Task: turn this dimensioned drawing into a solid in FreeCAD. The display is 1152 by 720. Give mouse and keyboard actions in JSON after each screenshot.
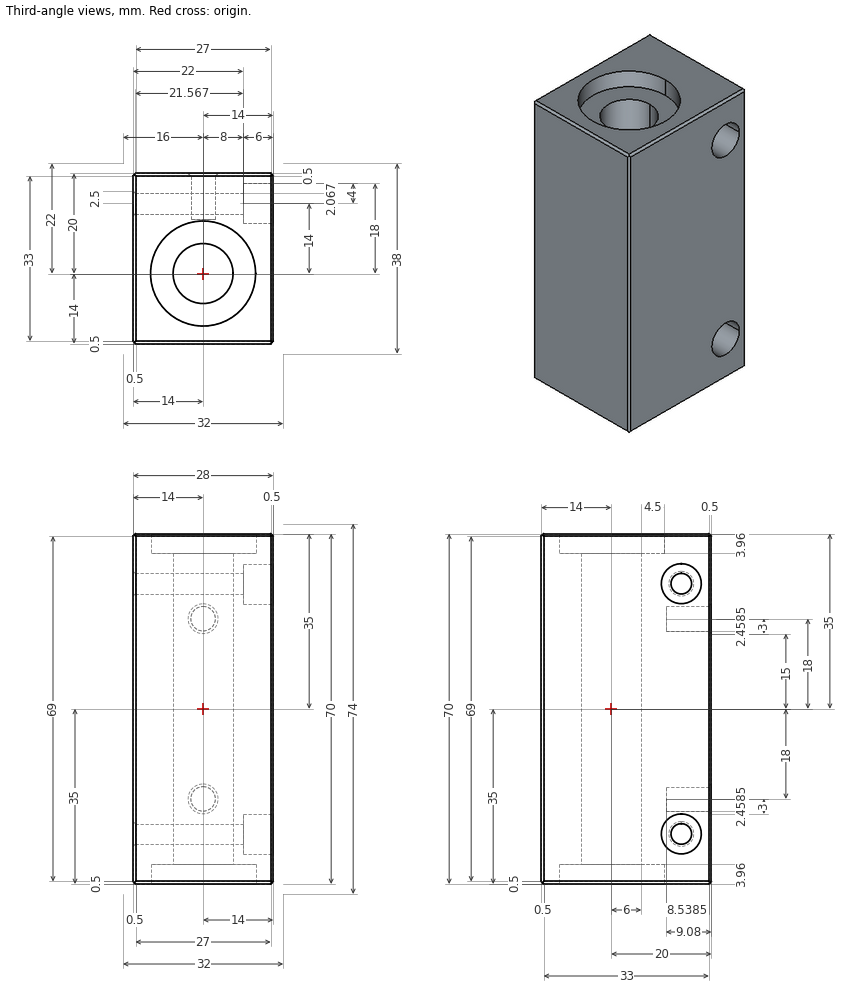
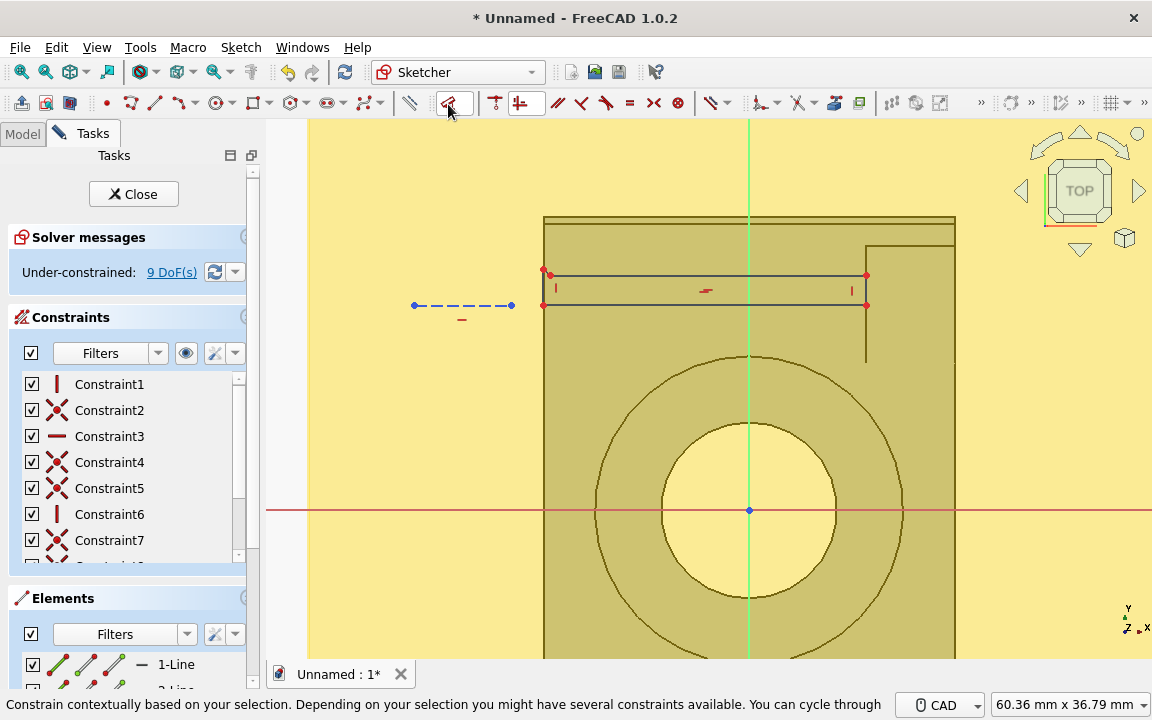
{"action": "left_click", "coordinate": [640, 305]}
{"action": "left_click", "coordinate": [705, 339]}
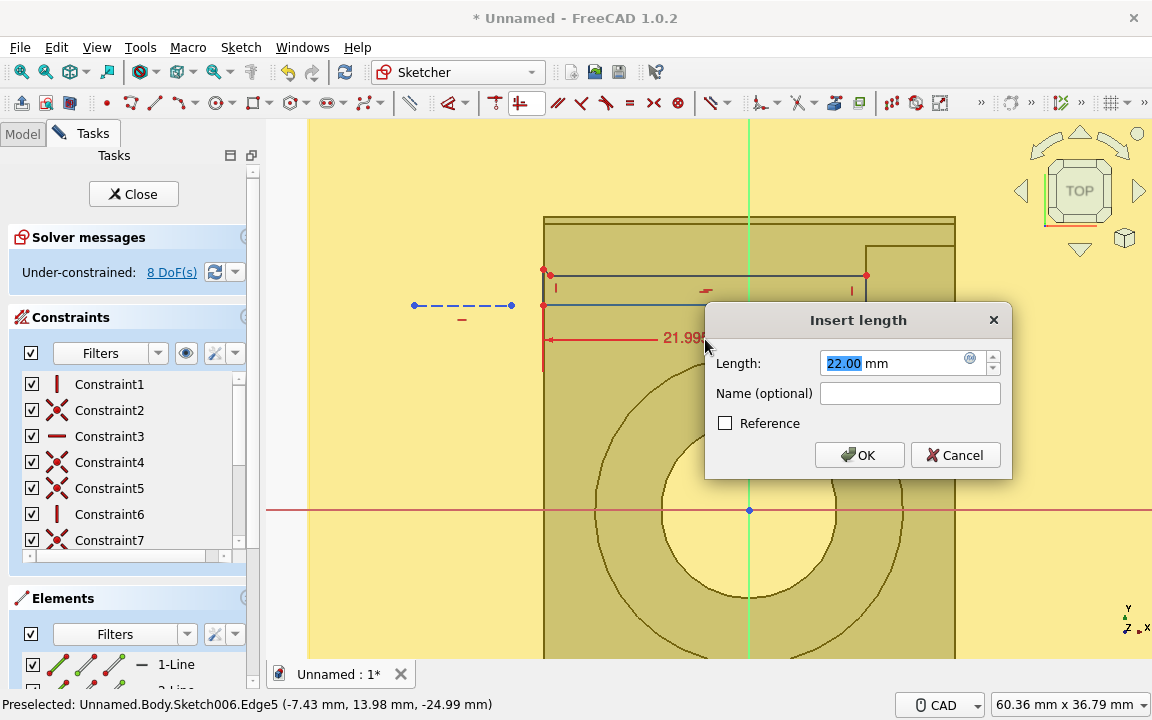
{"action": "type", "text": "22"}
{"action": "key", "text": "Return"}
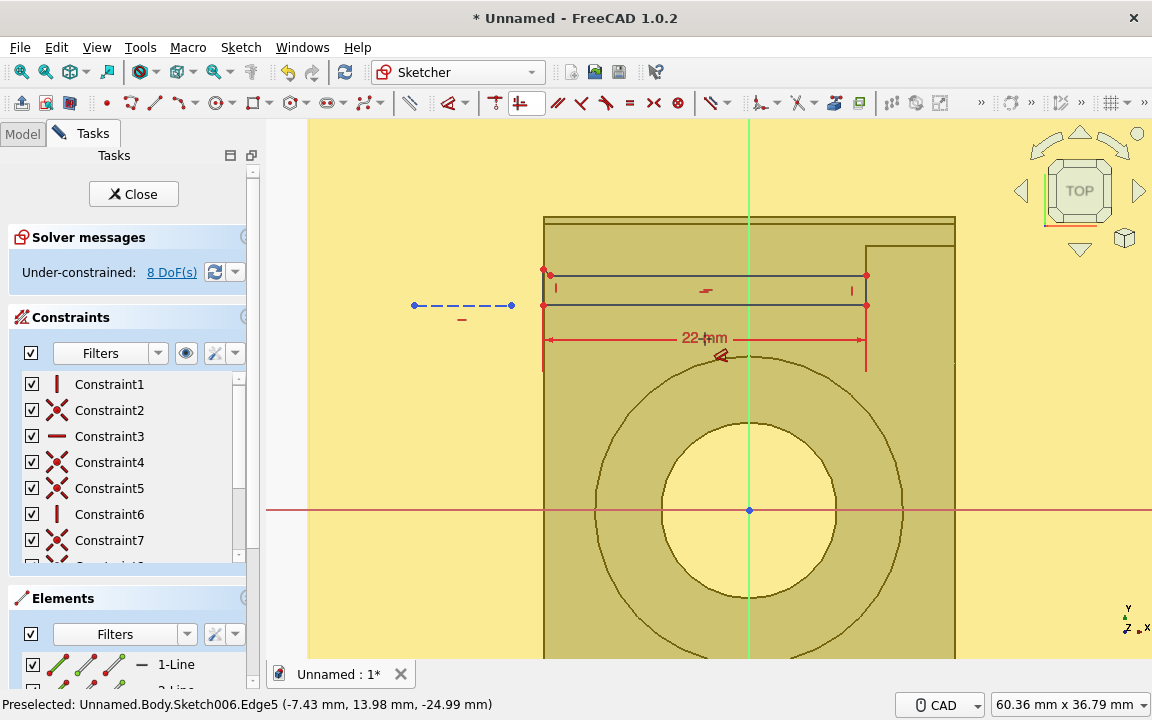
{"action": "left_click", "coordinate": [866, 305]}
{"action": "left_click", "coordinate": [808, 544]}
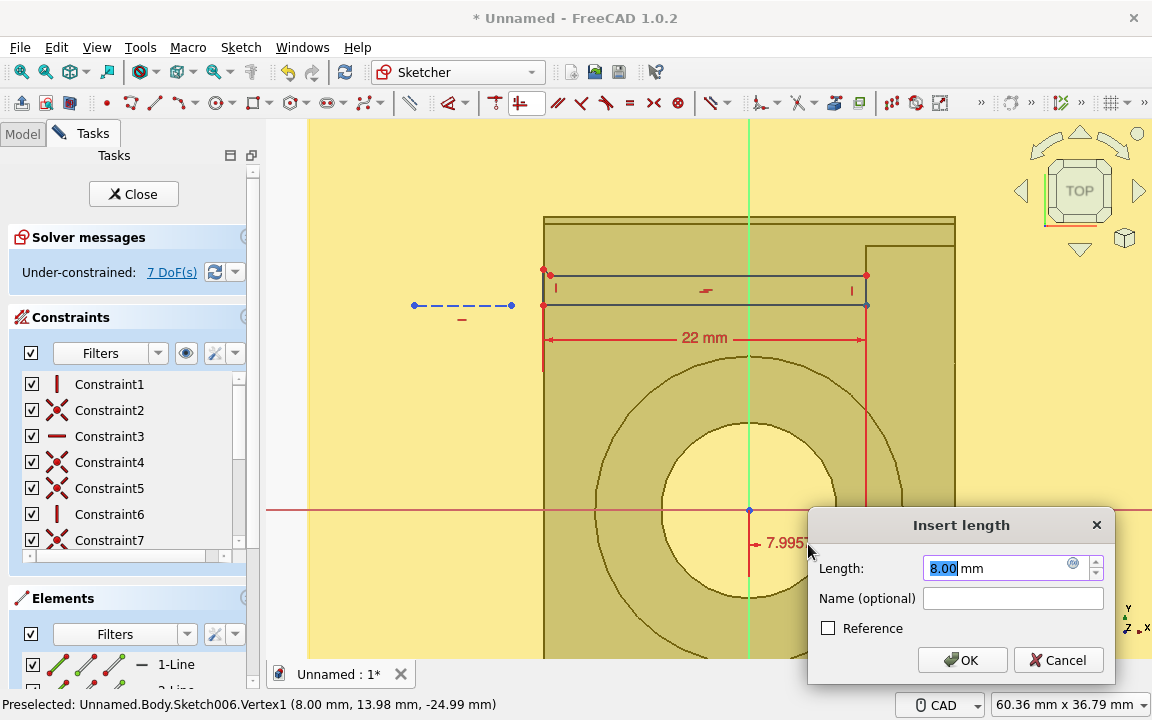
{"action": "type", "text": "8"}
{"action": "key", "text": "Return"}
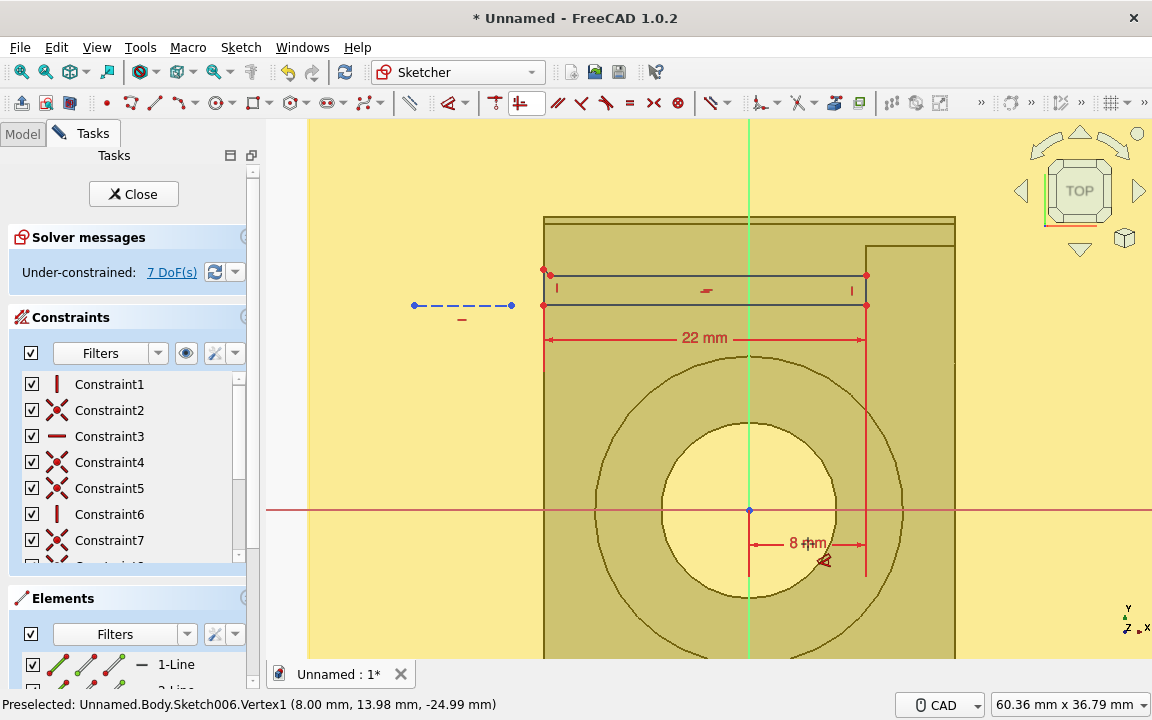
{"action": "scroll", "coordinate": [544, 294], "scroll_direction": "up", "scroll_amount": 2}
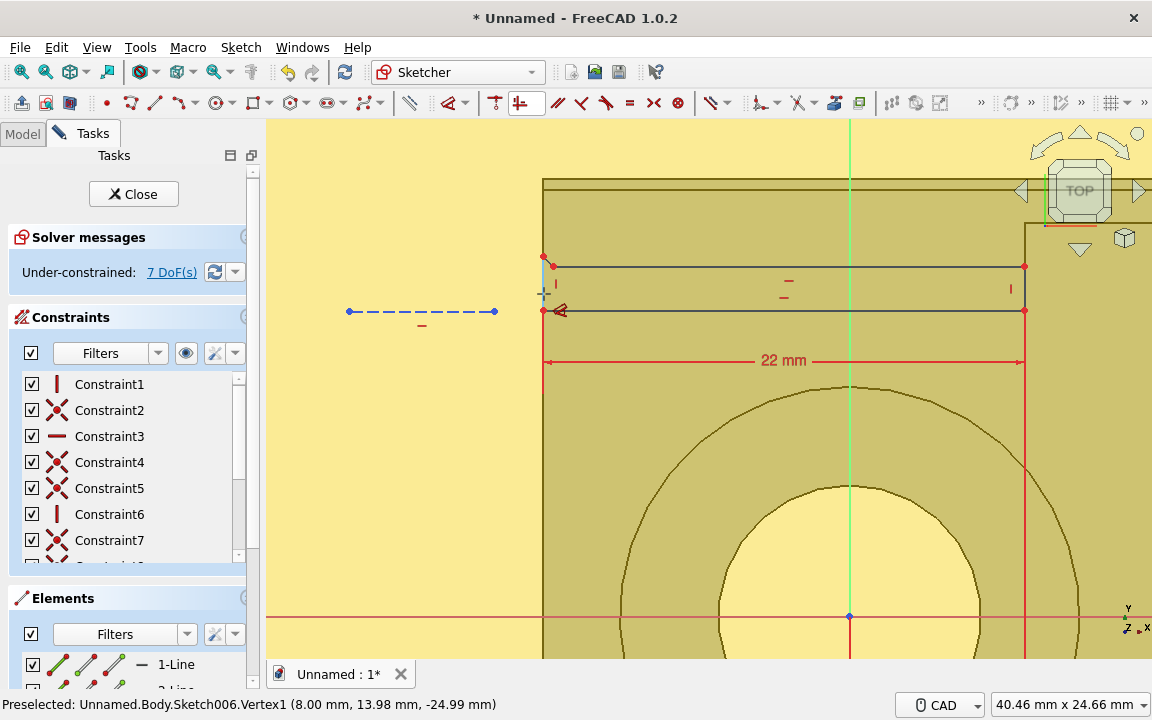
{"action": "left_click", "coordinate": [543, 294]}
{"action": "left_click", "coordinate": [509, 284]}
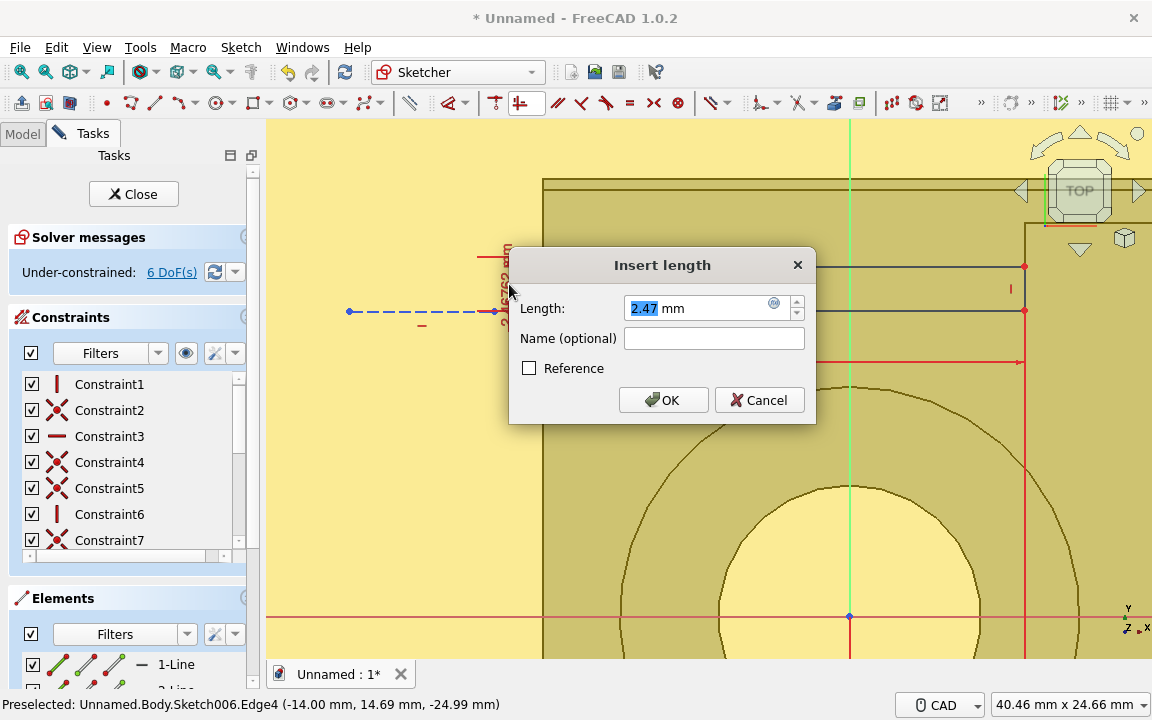
{"action": "type", "text": "2.5"}
{"action": "key", "text": "Return"}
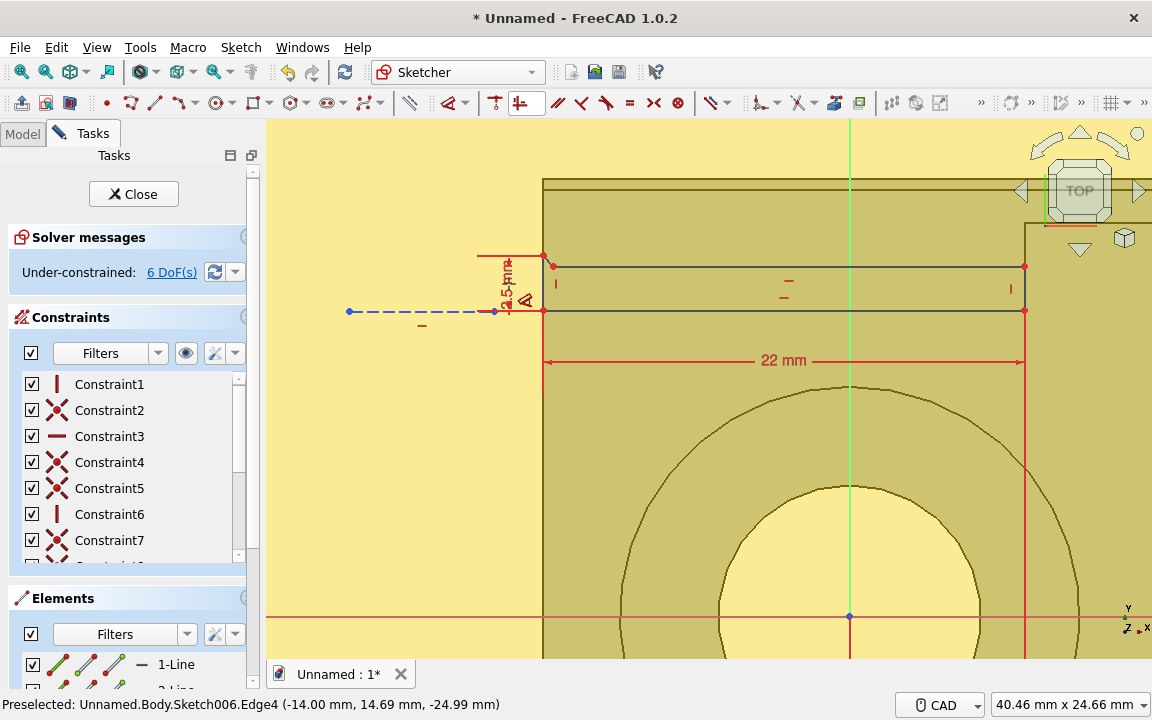
{"action": "scroll", "coordinate": [545, 293], "scroll_direction": "down", "scroll_amount": 2}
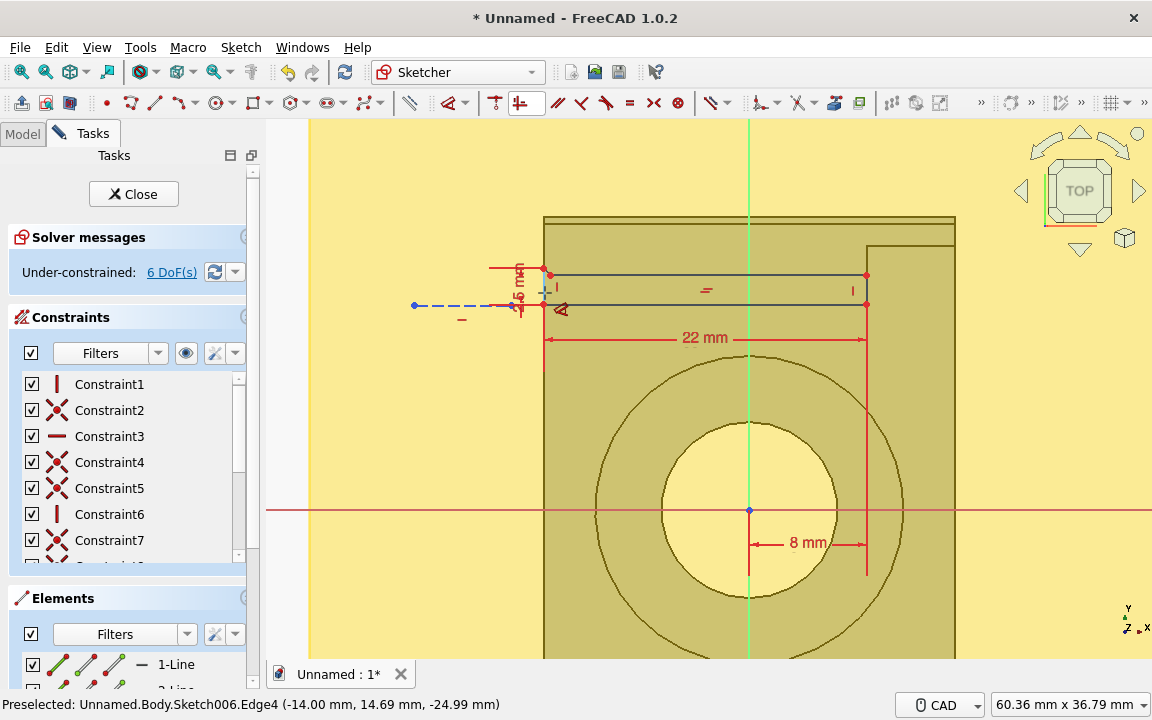
{"action": "left_click", "coordinate": [867, 305]}
{"action": "left_click", "coordinate": [901, 408]}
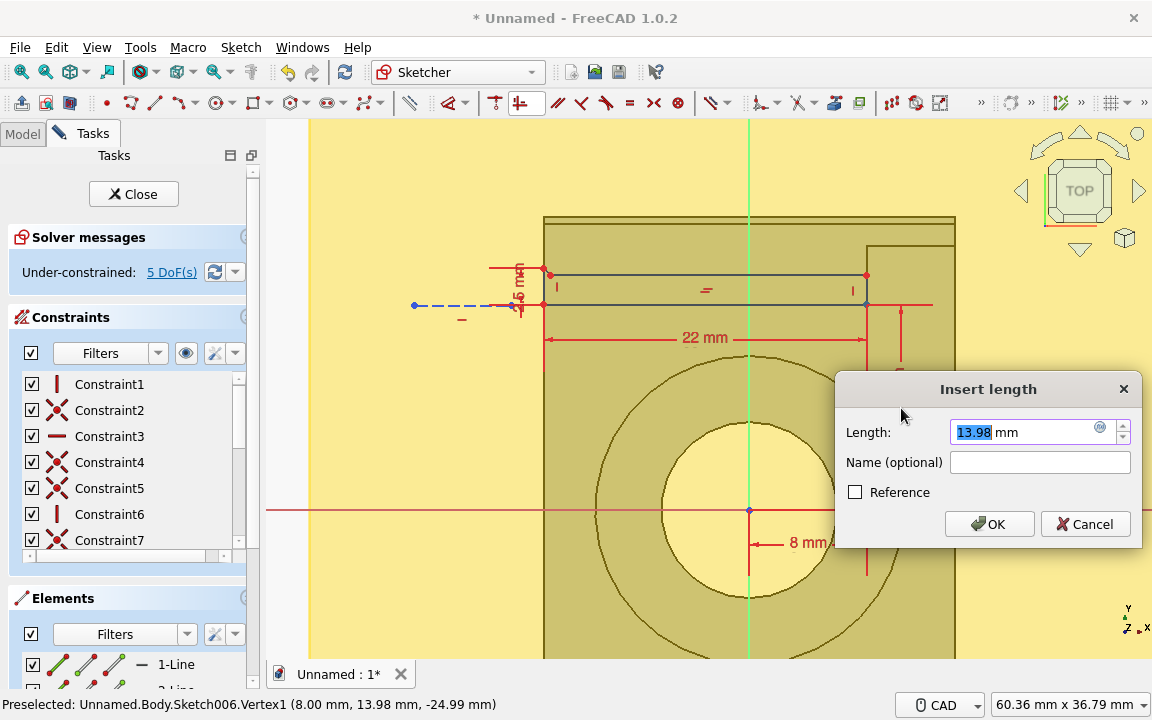
{"action": "type", "text": "14"}
{"action": "key", "text": "Return"}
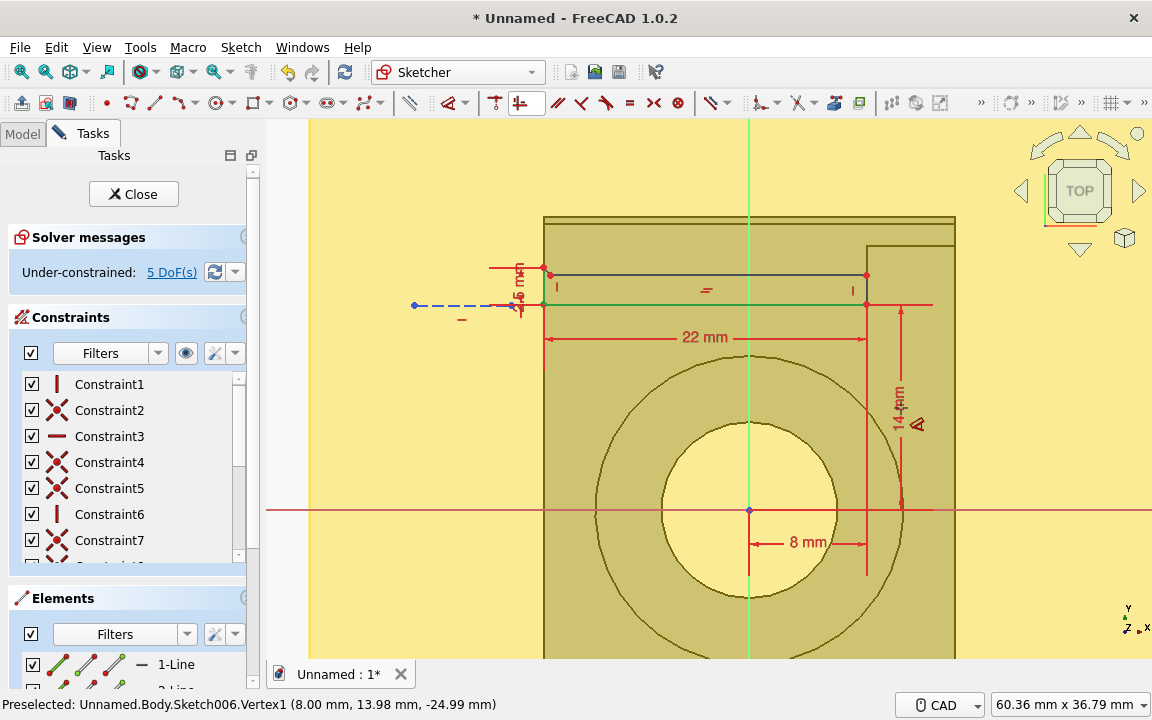
{"action": "left_click", "coordinate": [511, 306]}
{"action": "left_click", "coordinate": [477, 408]}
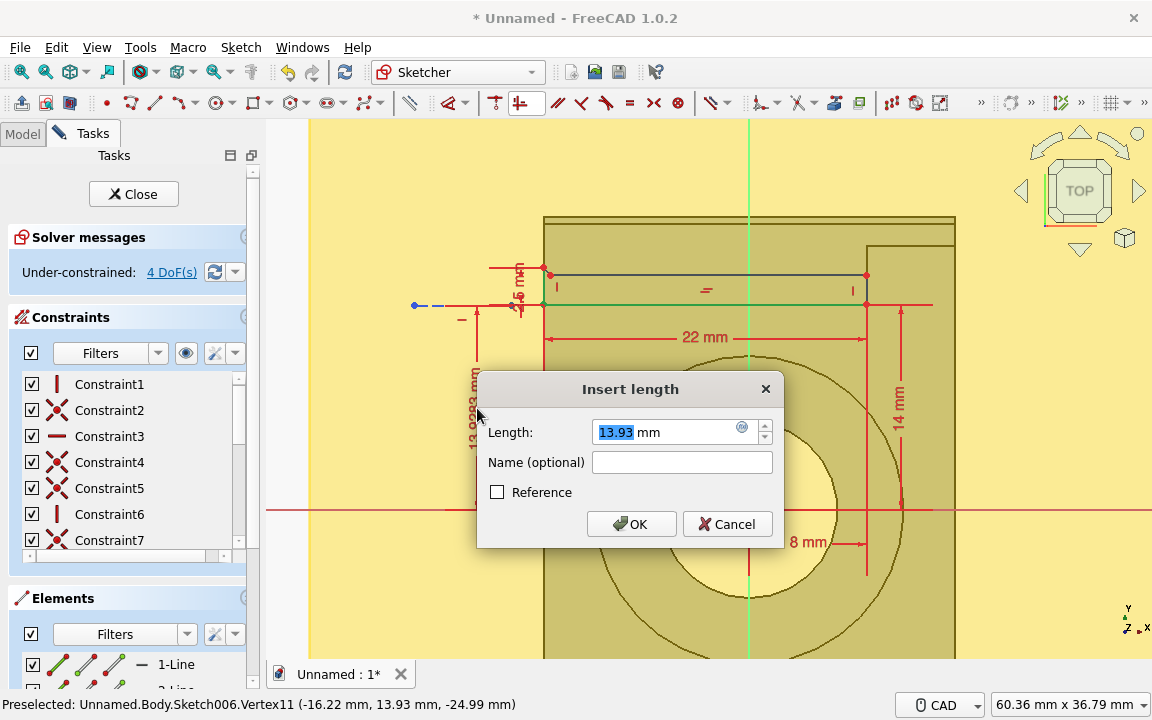
{"action": "type", "text": "14"}
{"action": "key", "text": "Return"}